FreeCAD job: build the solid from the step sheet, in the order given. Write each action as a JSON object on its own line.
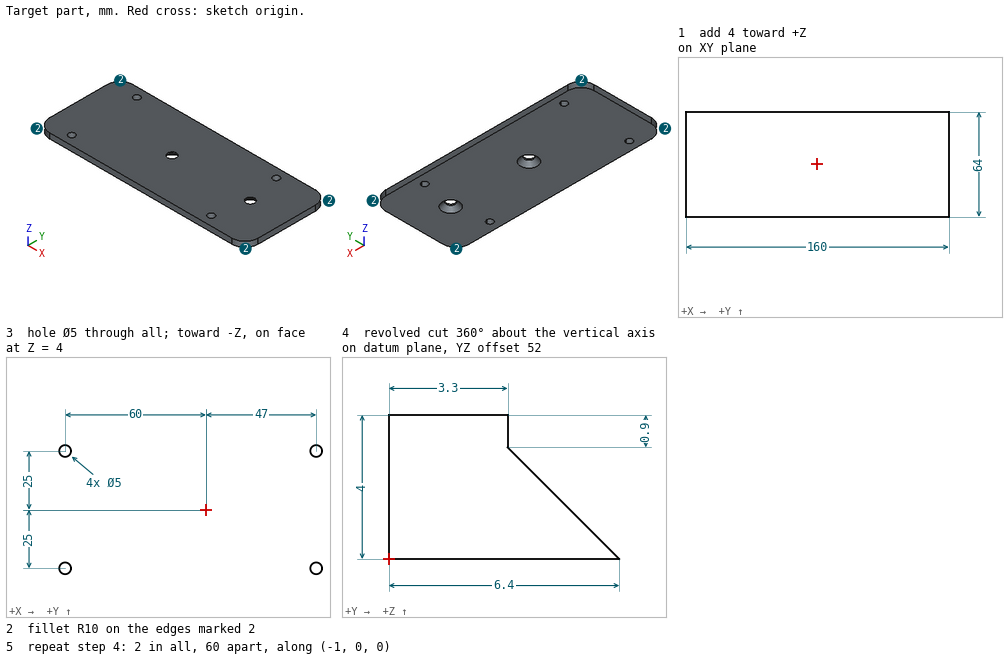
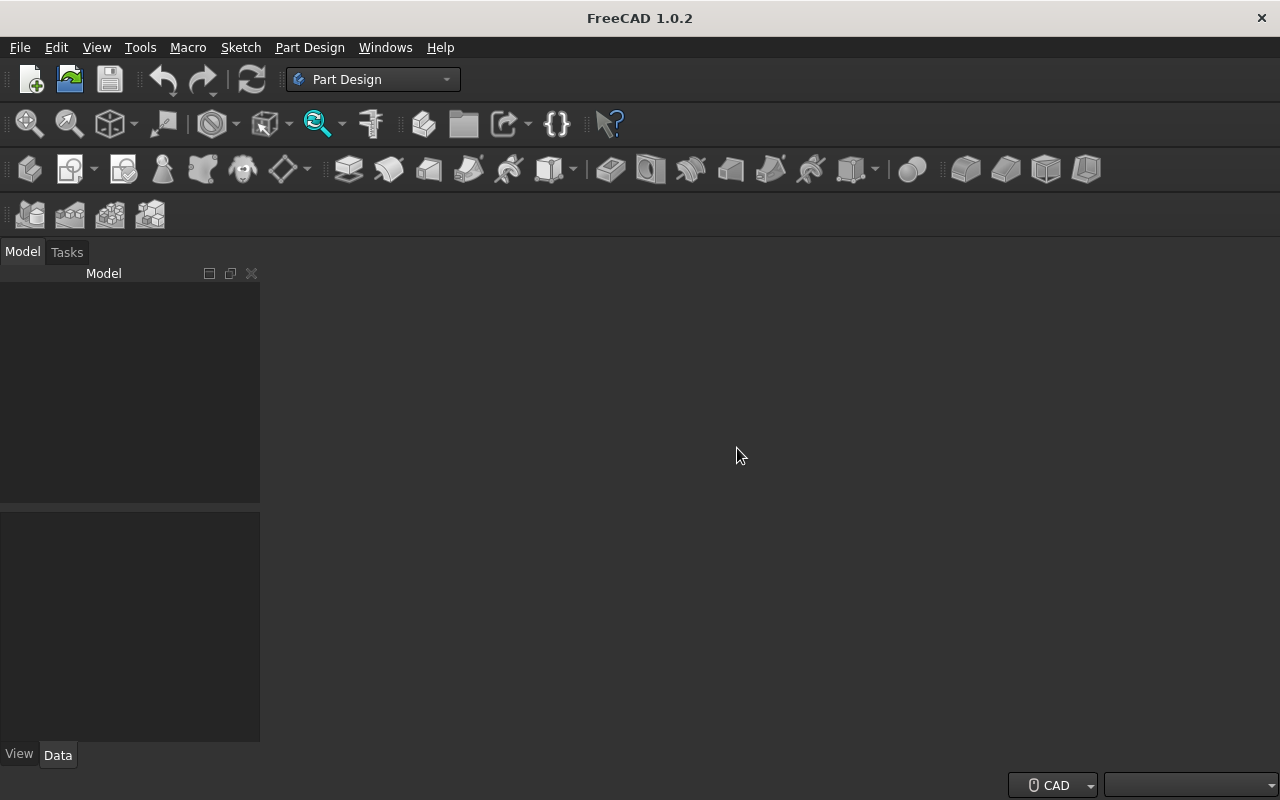
{"action": "left_click", "coordinate": [30, 80]}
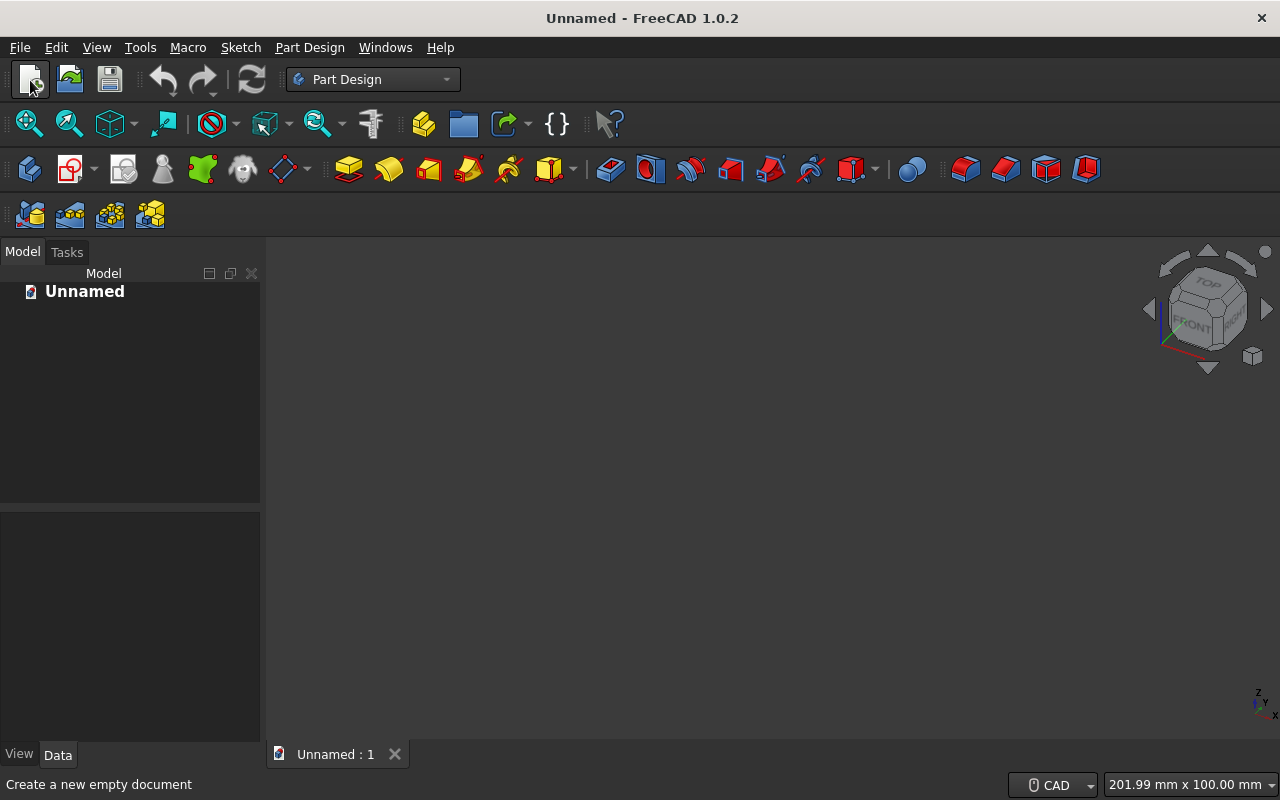
{"action": "left_click", "coordinate": [70, 170]}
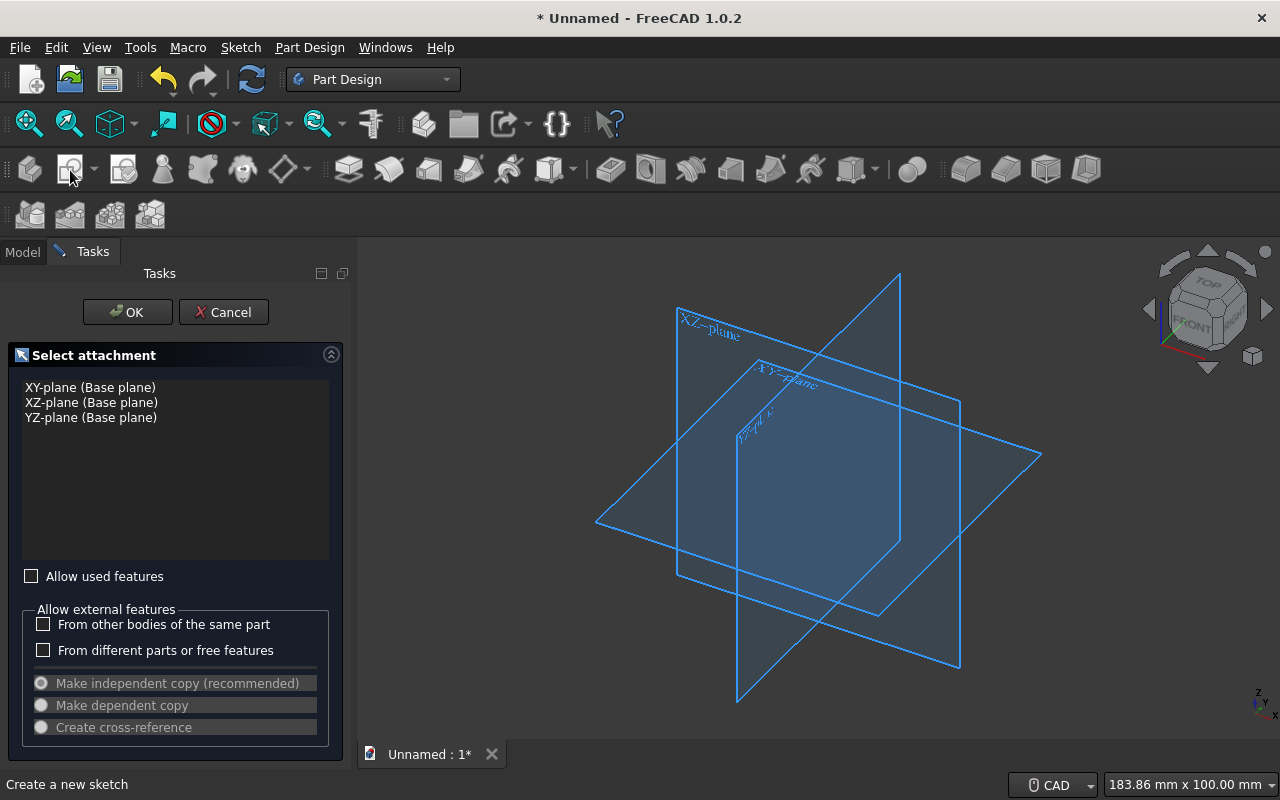
{"action": "left_click", "coordinate": [82, 388]}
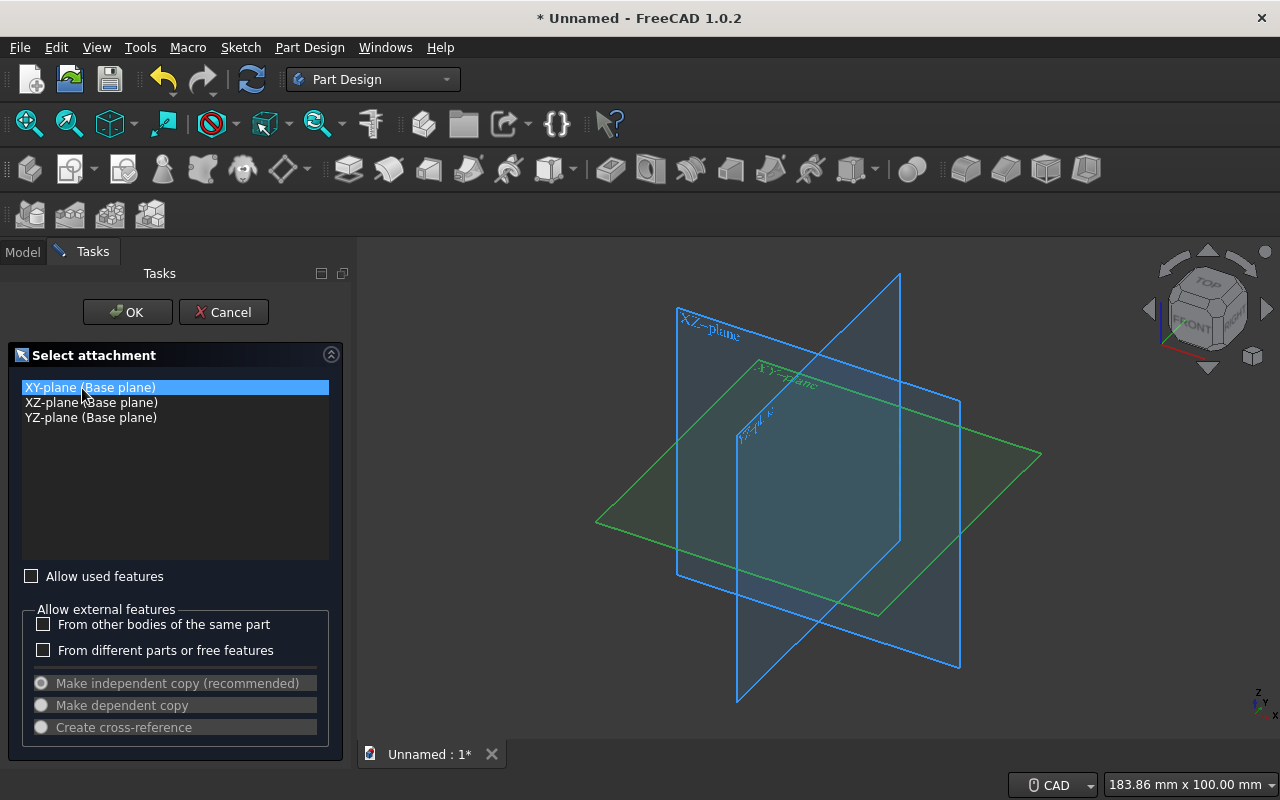
{"action": "left_click", "coordinate": [128, 312]}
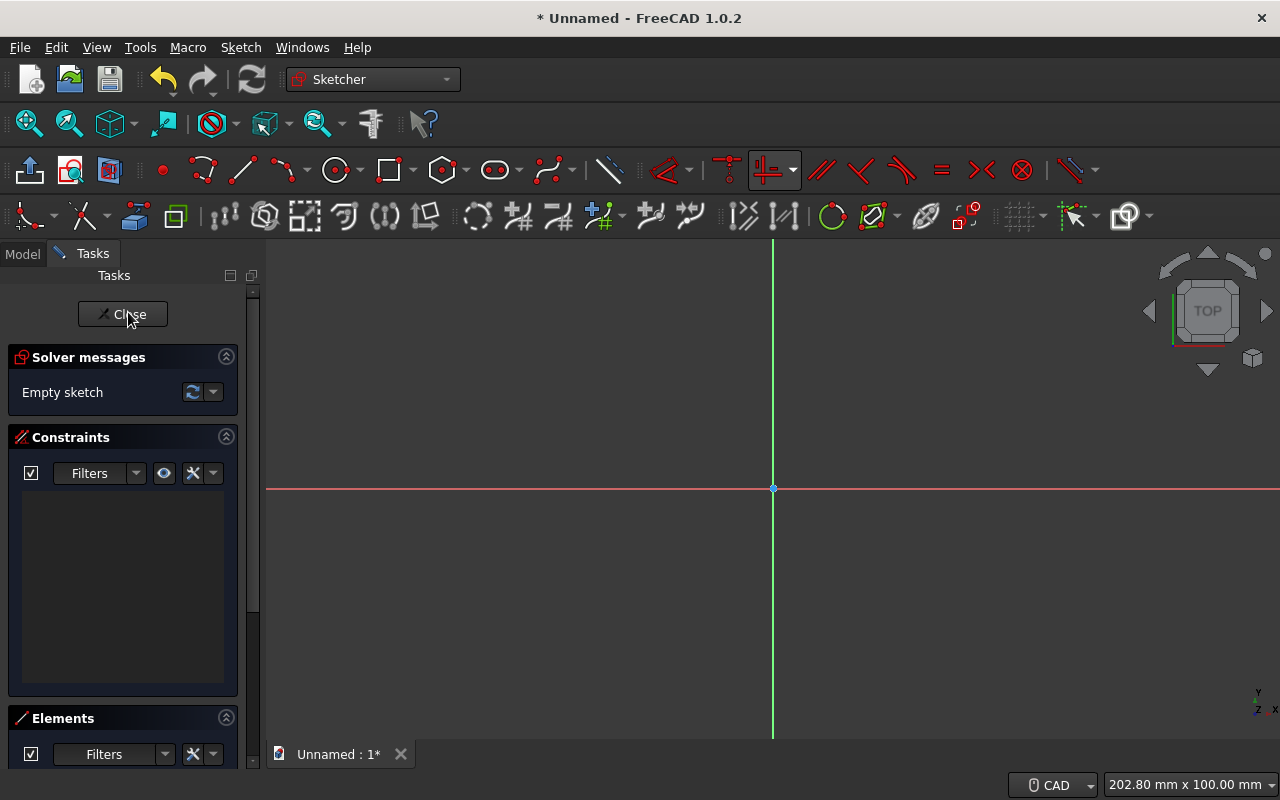
{"action": "scroll", "coordinate": [565, 489], "scroll_direction": "down", "scroll_amount": 2}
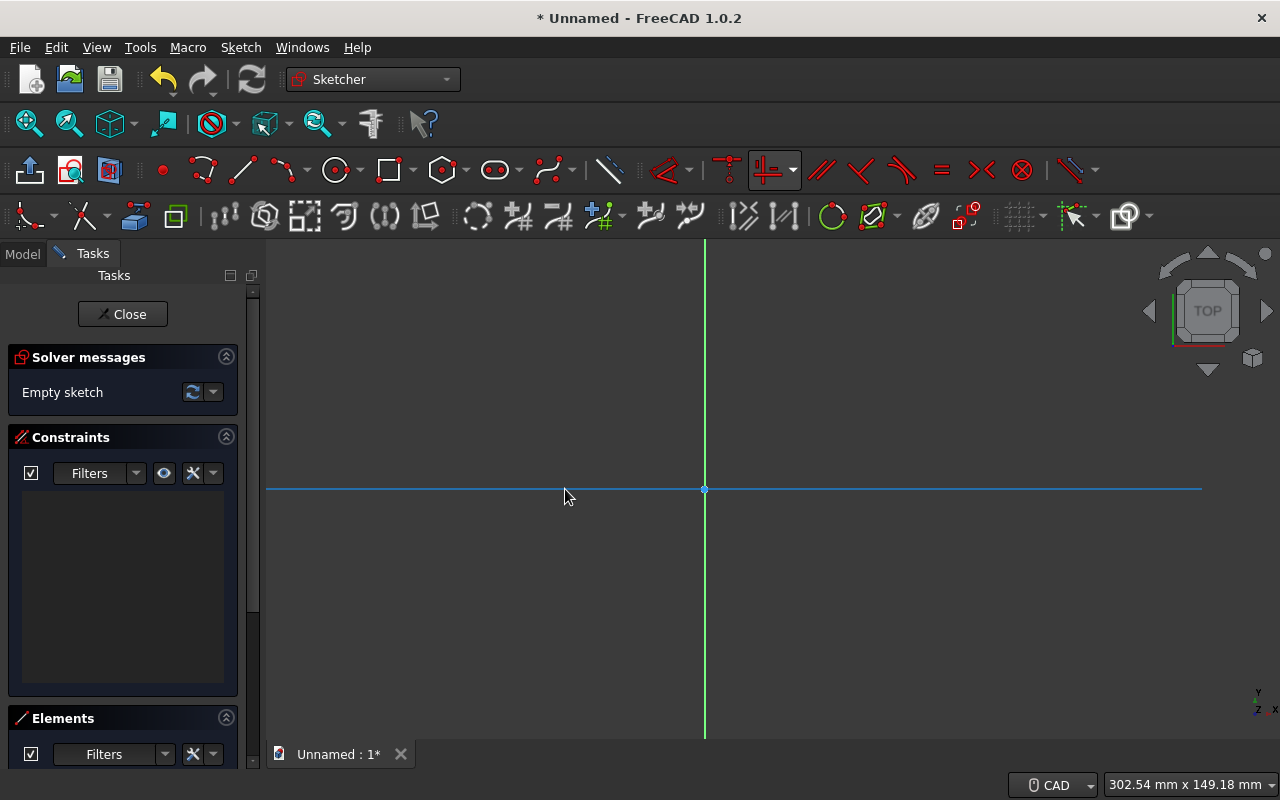
{"action": "left_click", "coordinate": [416, 170]}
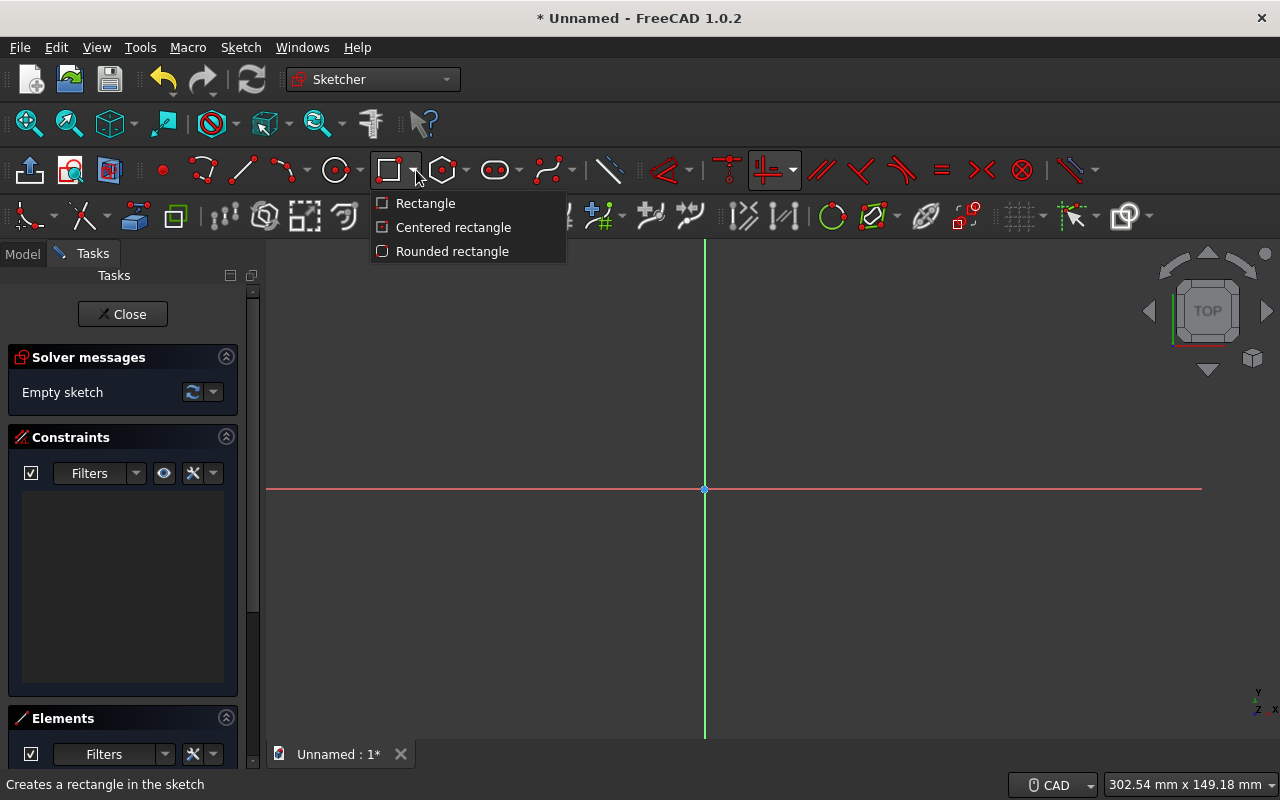
{"action": "left_click", "coordinate": [468, 227]}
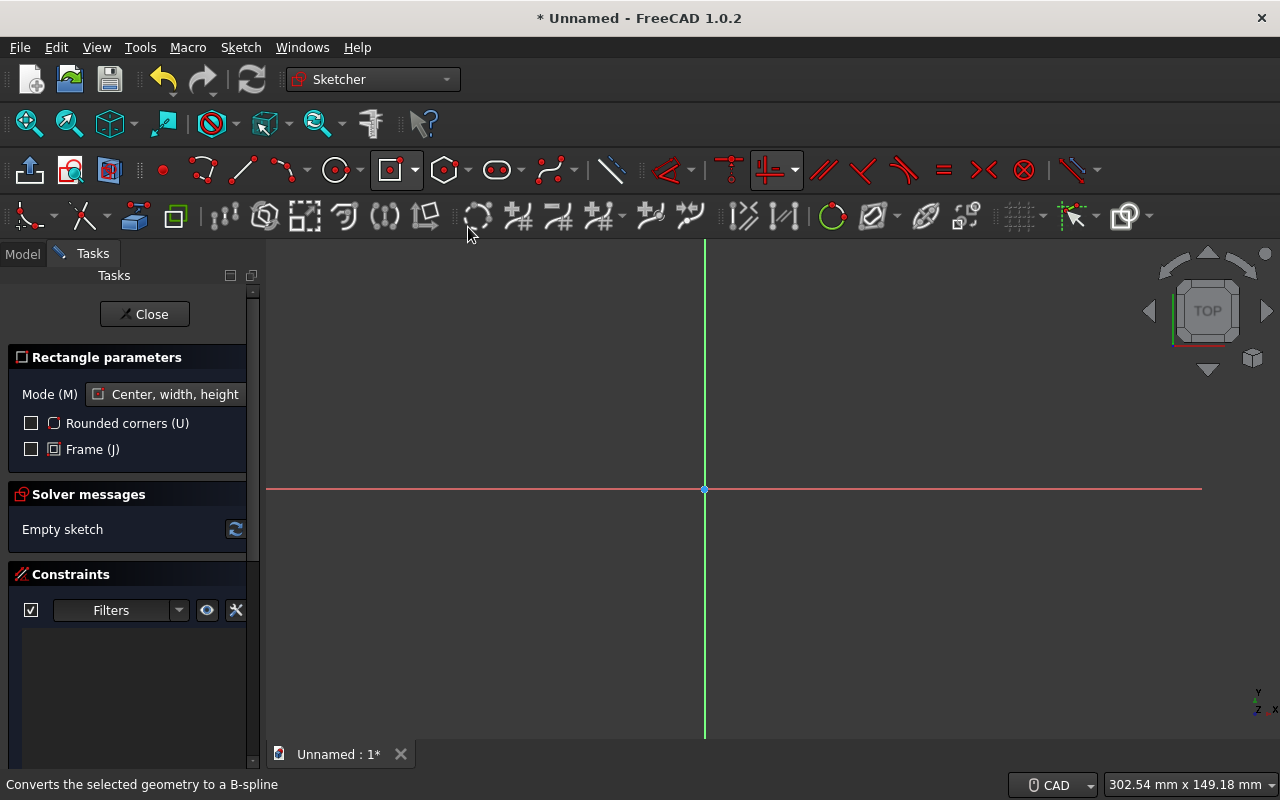
{"action": "left_click", "coordinate": [705, 489]}
{"action": "left_click", "coordinate": [973, 382]}
{"action": "key", "text": "Escape"}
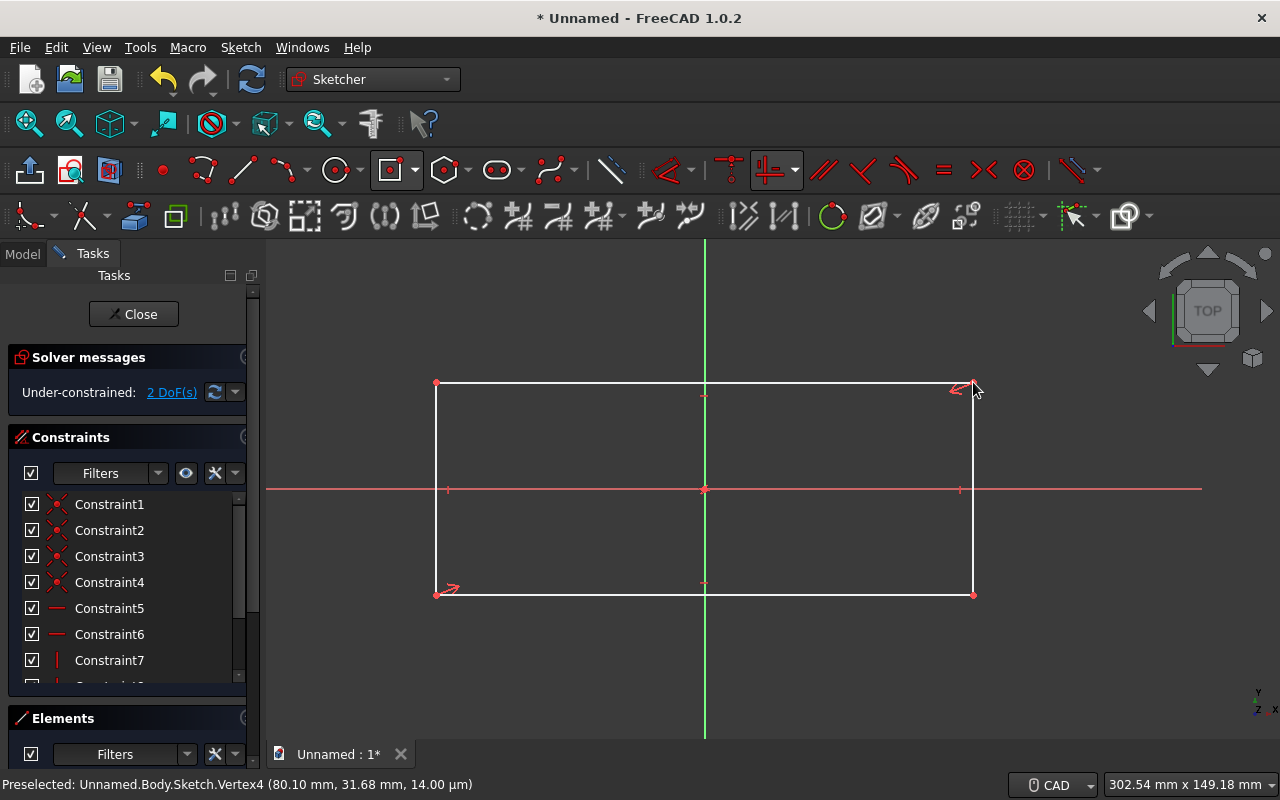
{"action": "left_click", "coordinate": [666, 170]}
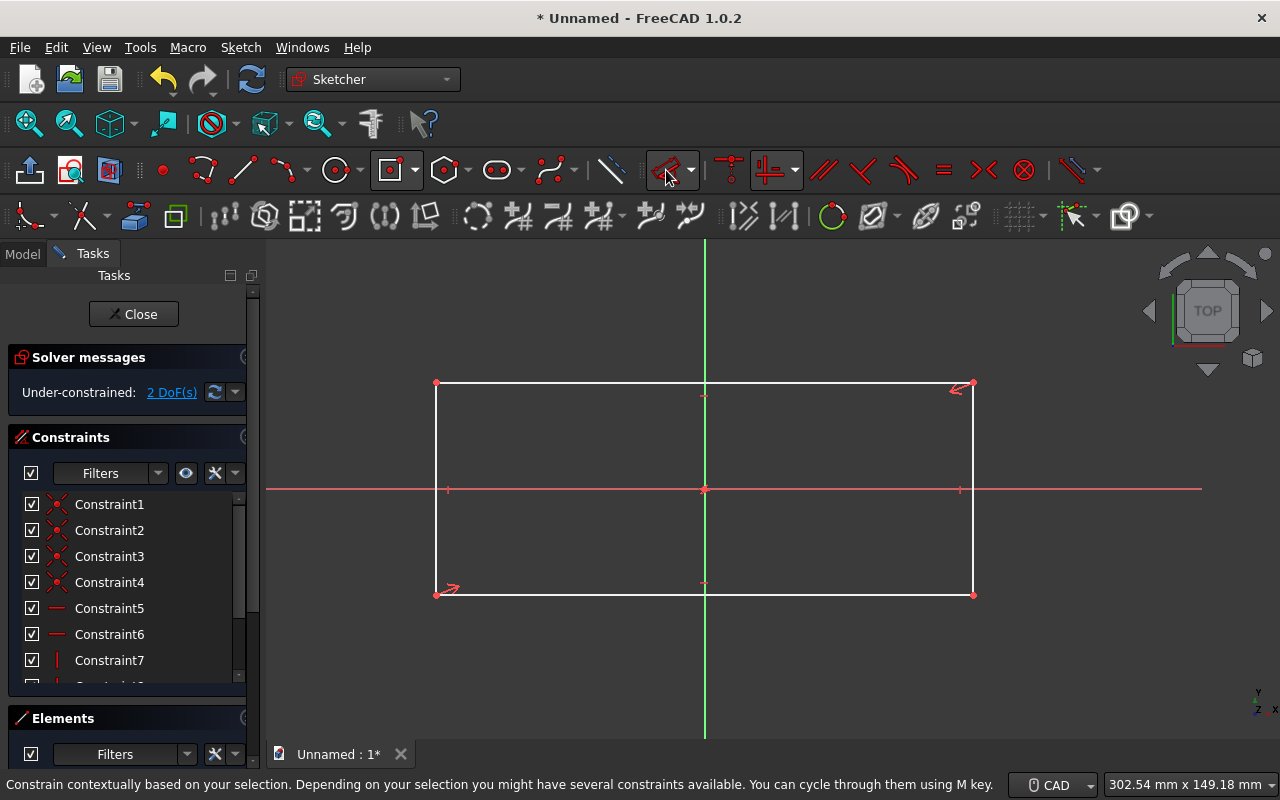
{"action": "left_click", "coordinate": [973, 532]}
{"action": "left_click", "coordinate": [1007, 440]}